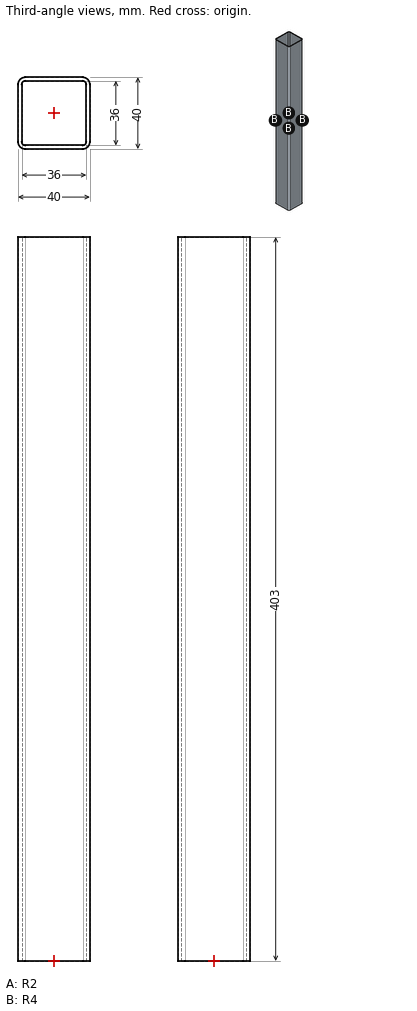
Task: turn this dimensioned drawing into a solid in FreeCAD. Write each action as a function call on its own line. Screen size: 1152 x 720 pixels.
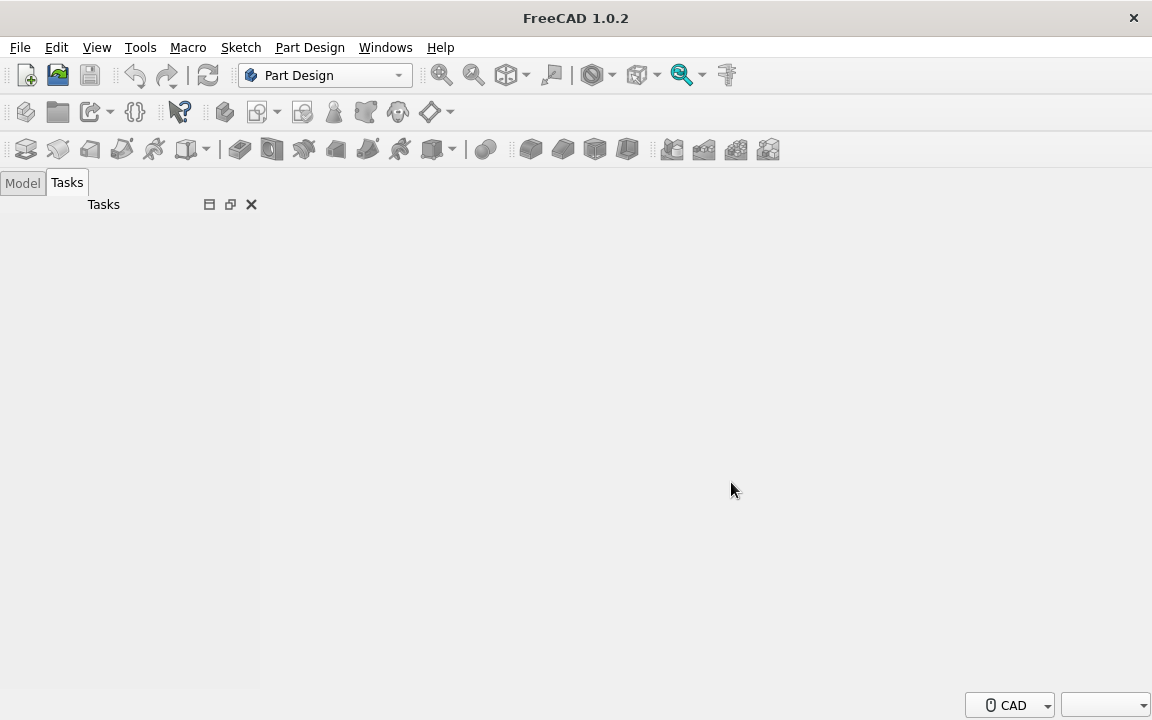
click(26, 76)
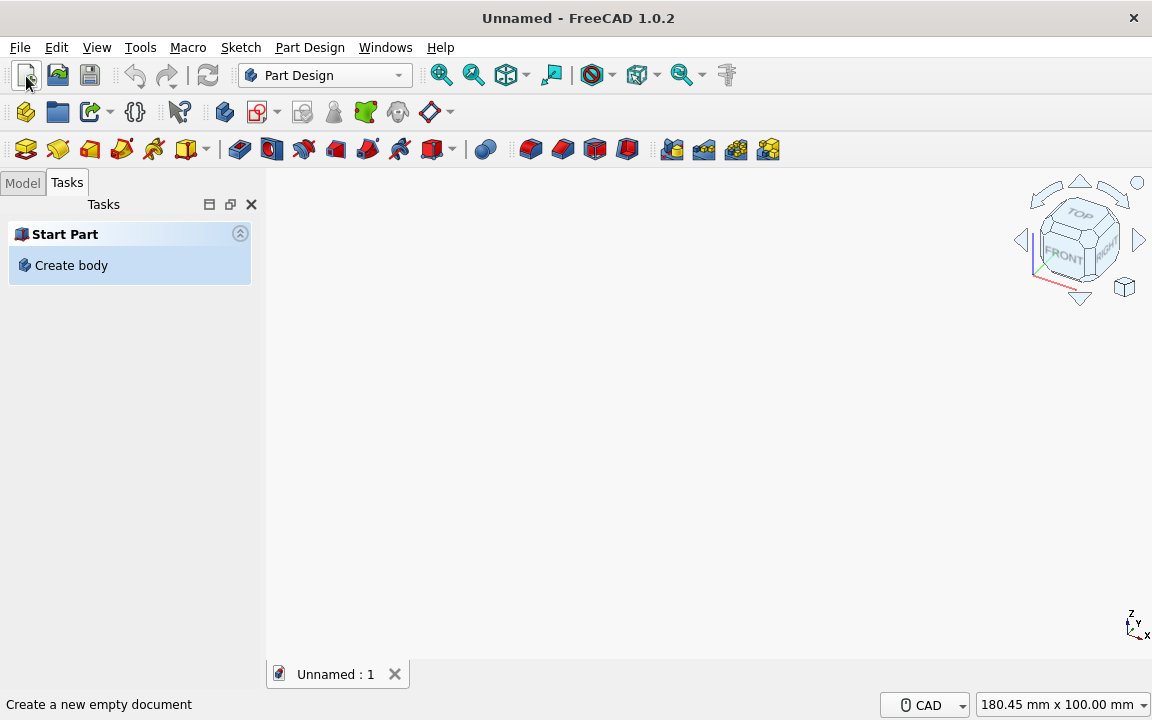
click(258, 112)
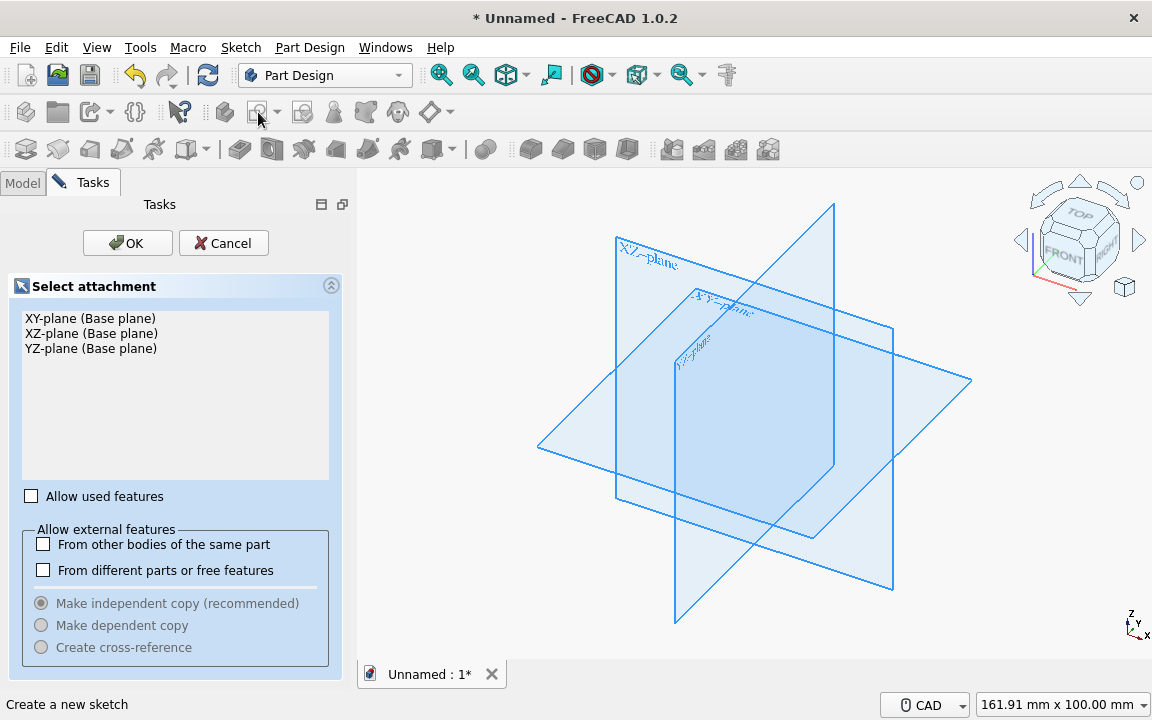
click(82, 318)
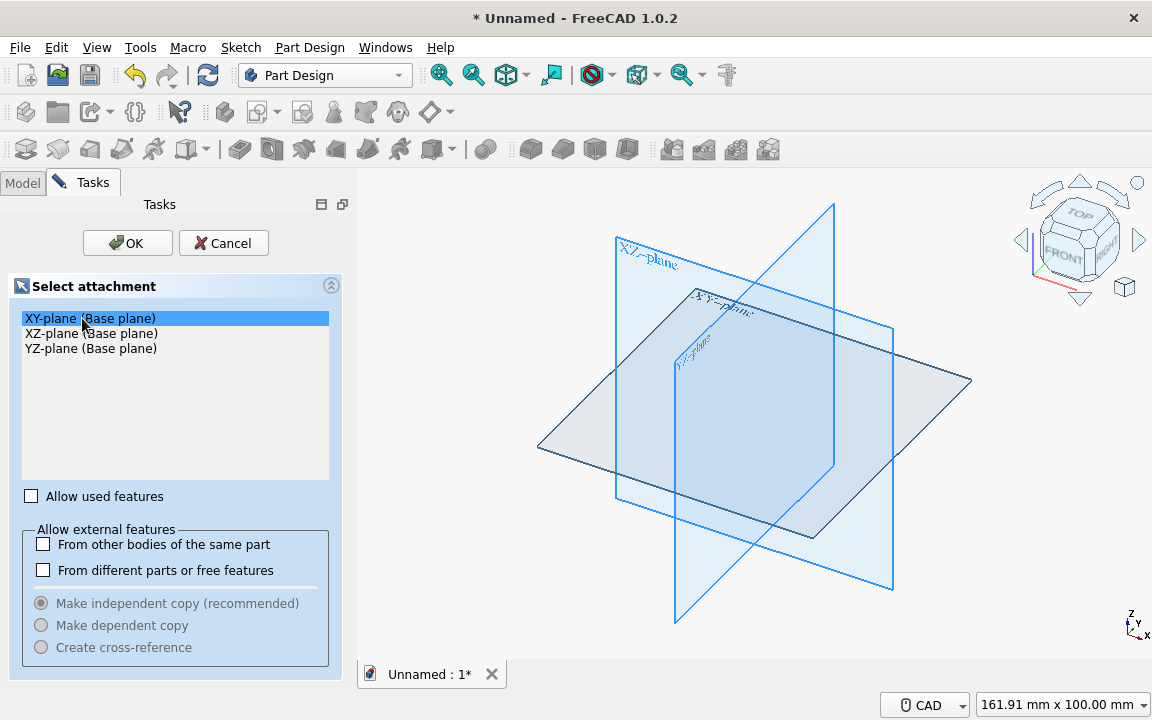
click(128, 243)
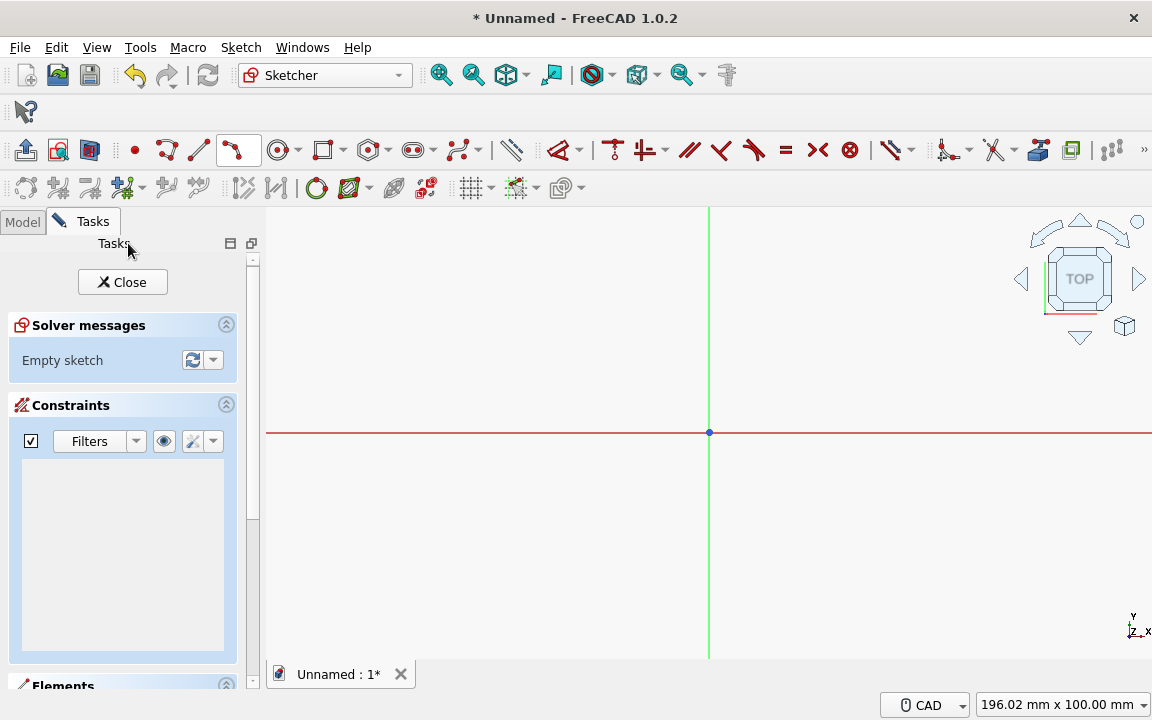
scroll(848, 433, up, 2)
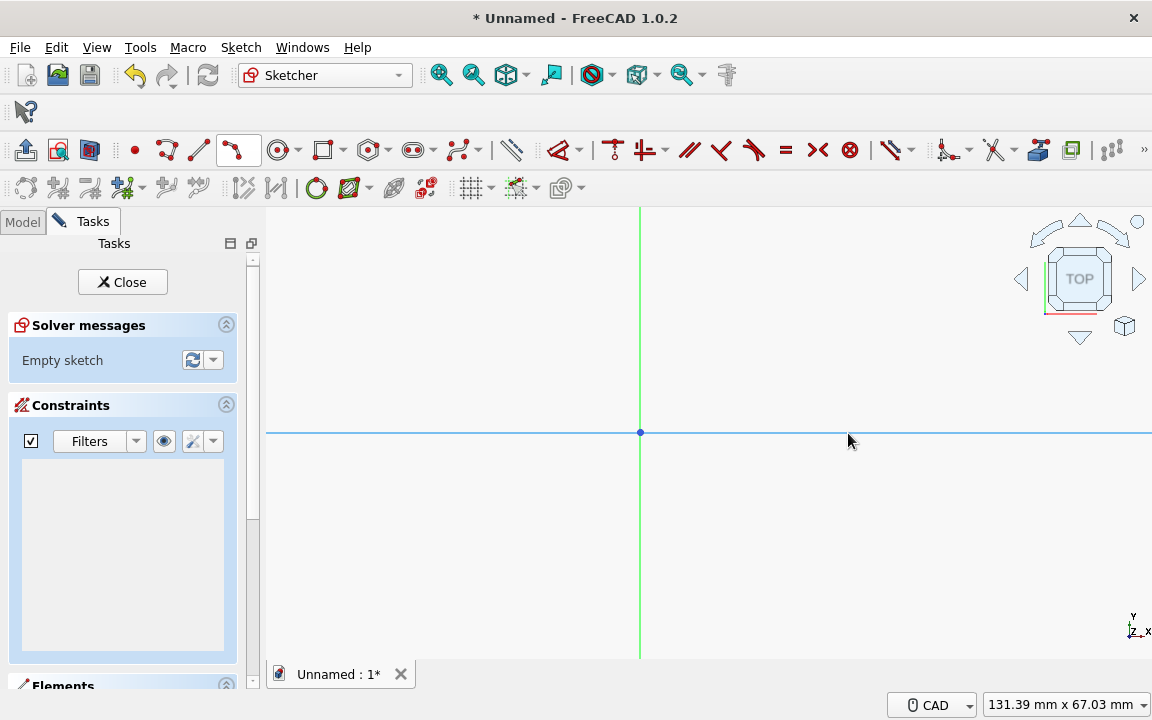
key(g)
key(v)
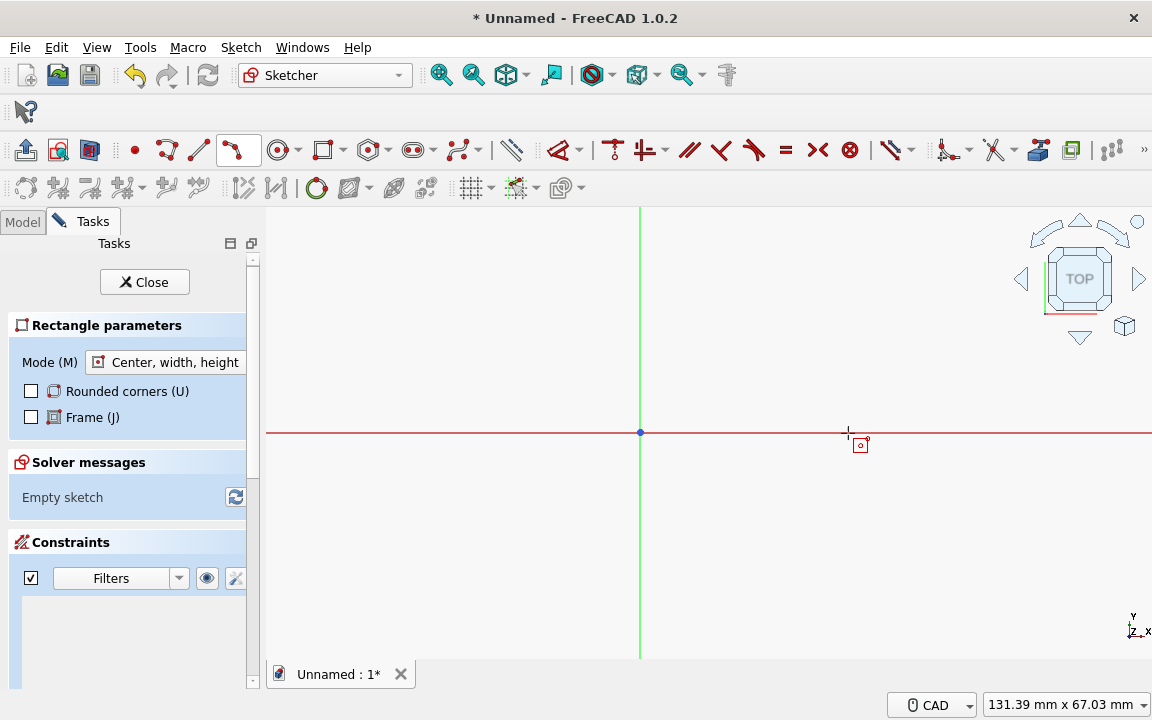
click(640, 433)
move(775, 298)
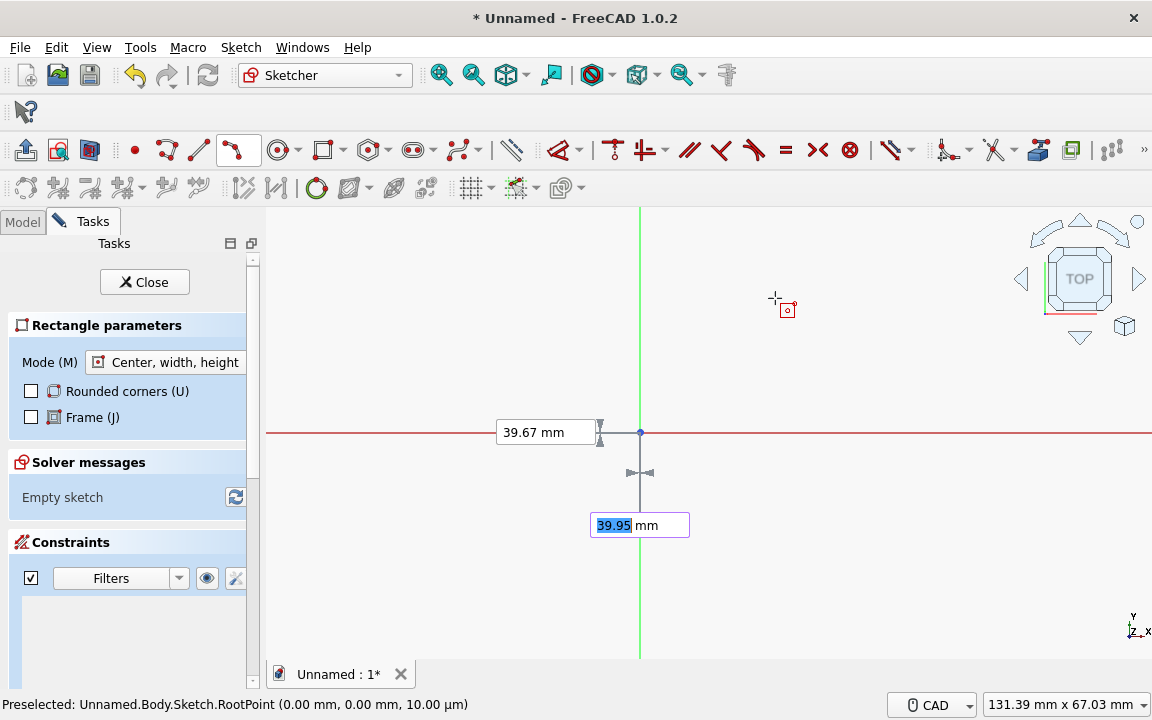
text(40)
key(Tab)
text(40)
key(Return)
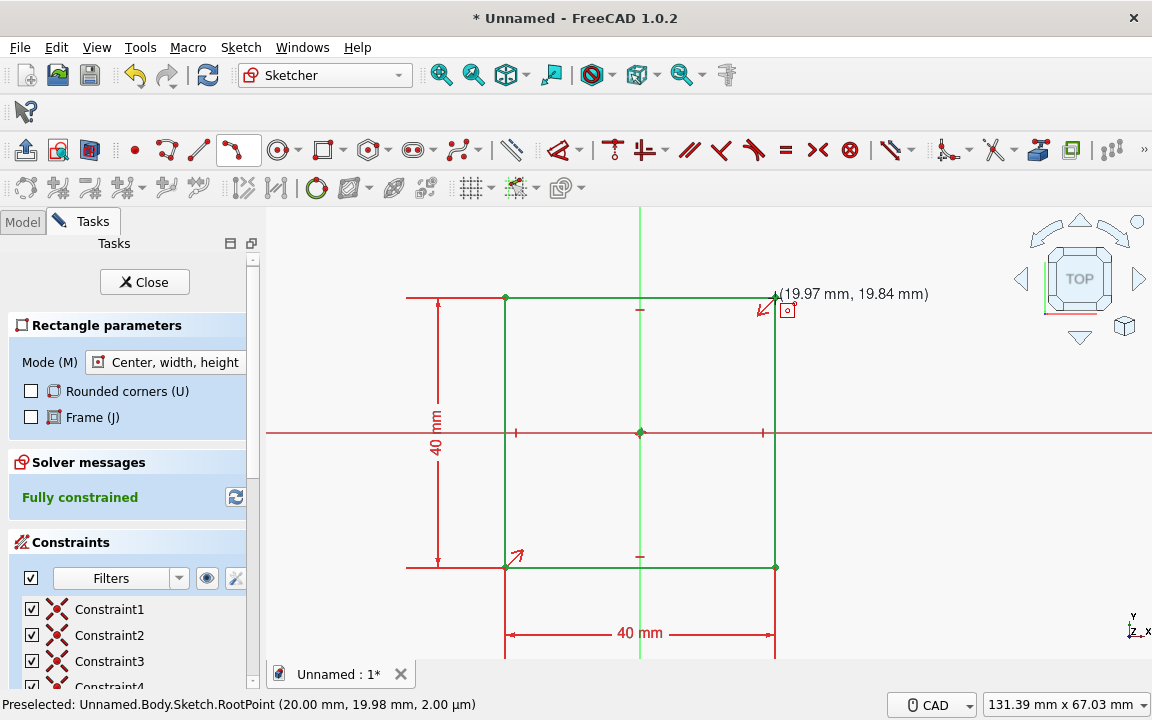
click(640, 433)
move(762, 311)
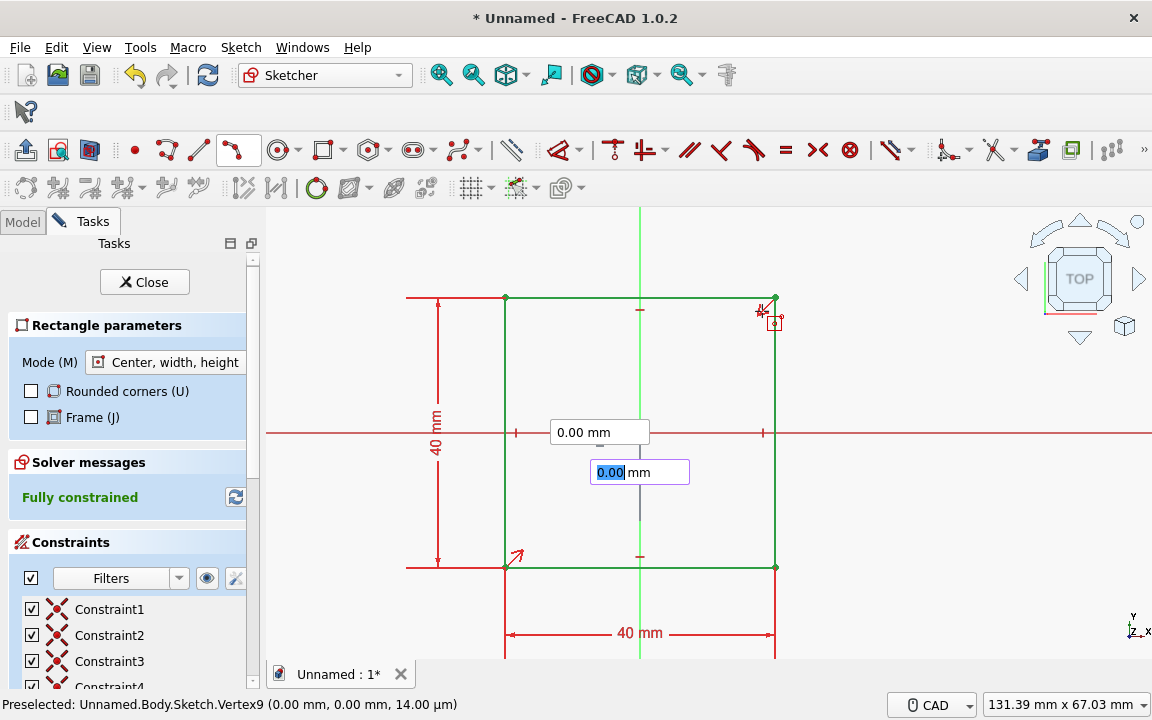
text(36)
key(Tab)
text(36)
key(Return)
key(Escape)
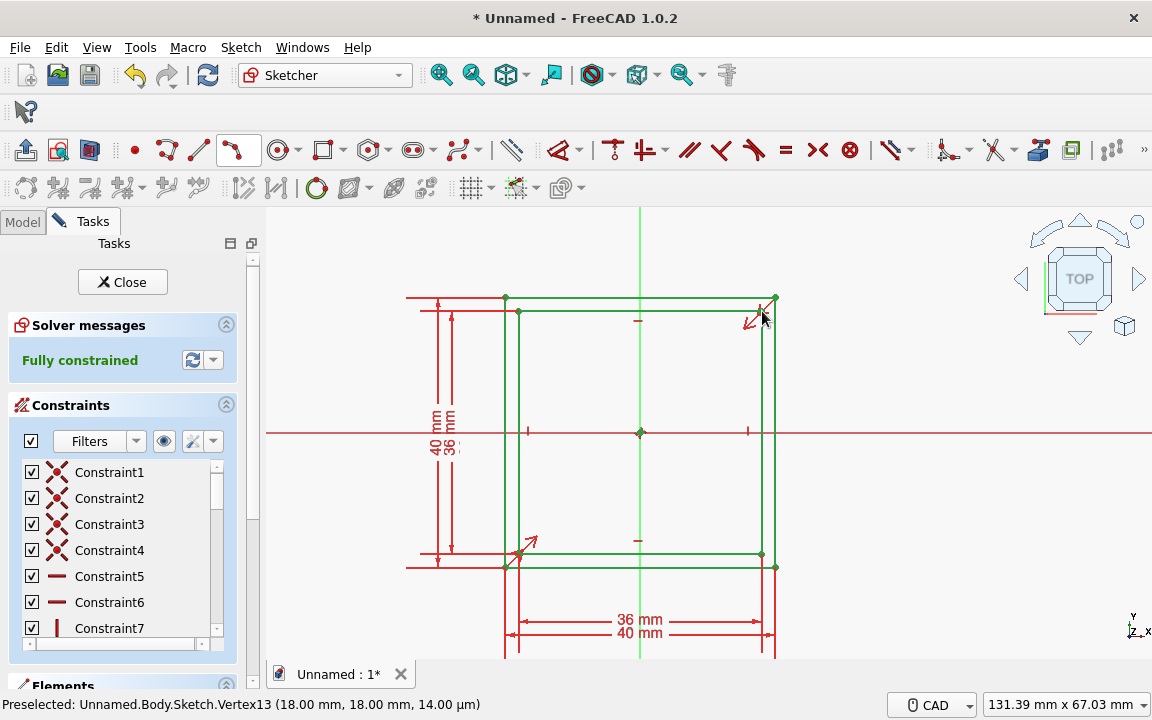
click(123, 282)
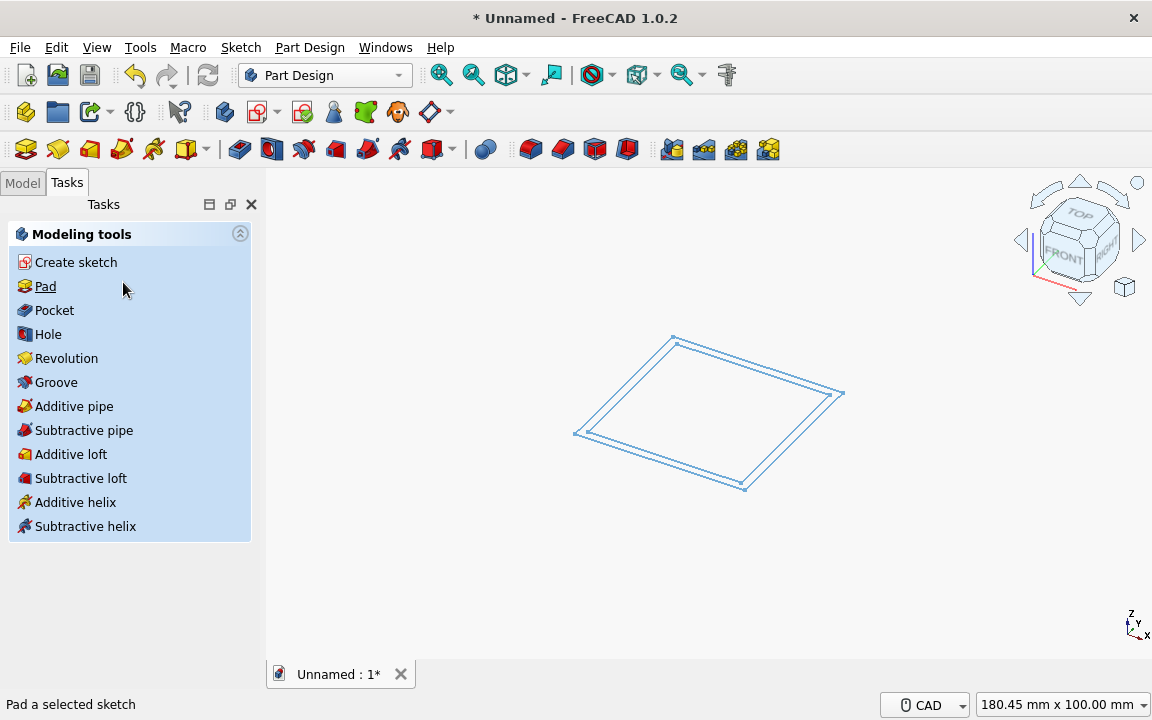
click(26, 150)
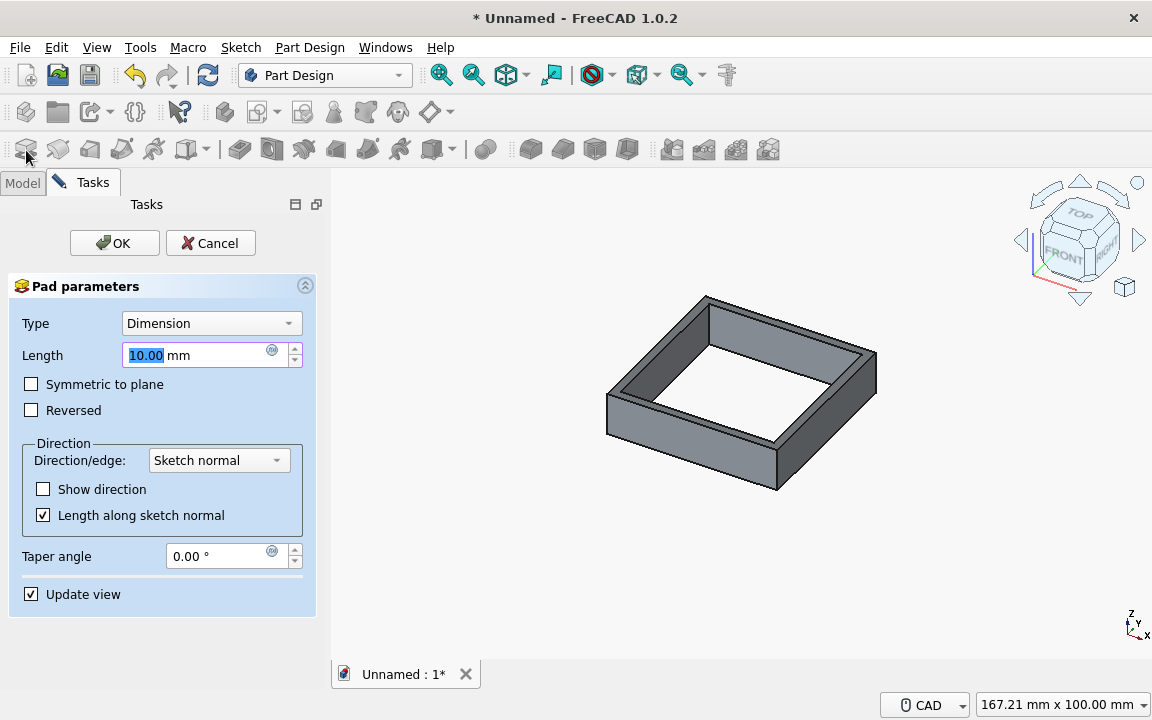
text(403)
key(Tab)